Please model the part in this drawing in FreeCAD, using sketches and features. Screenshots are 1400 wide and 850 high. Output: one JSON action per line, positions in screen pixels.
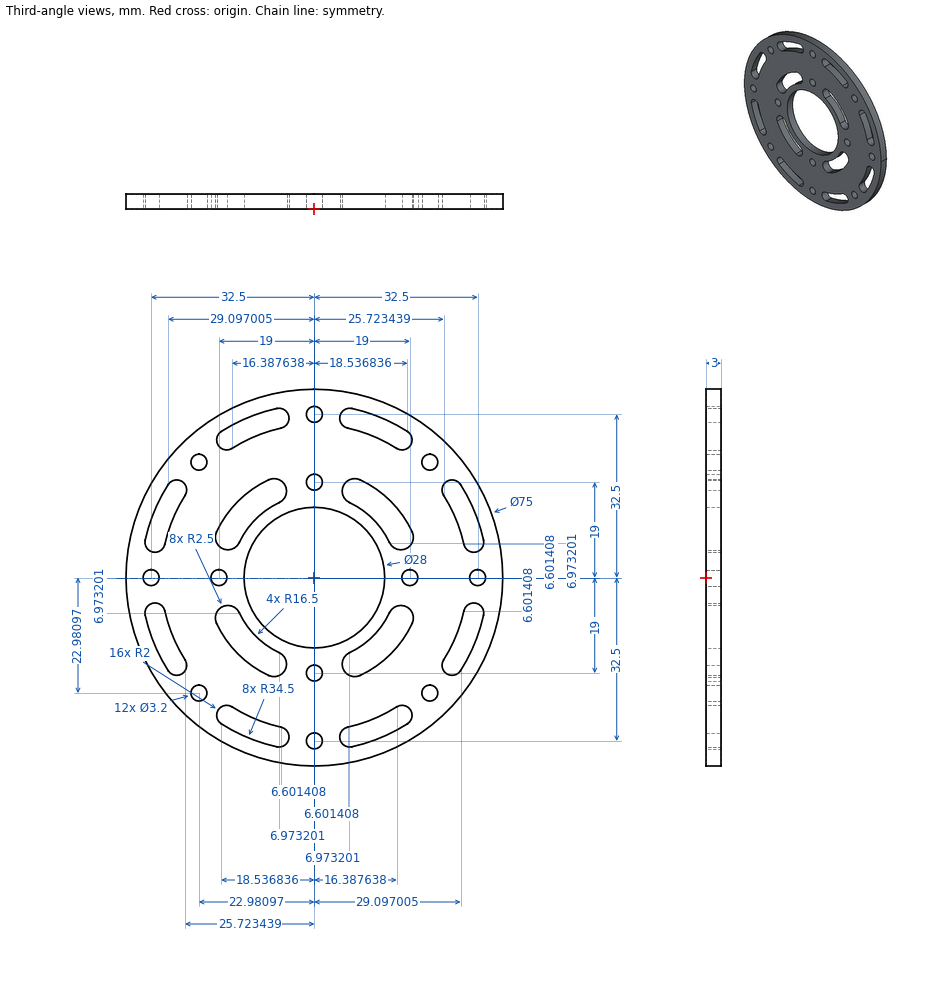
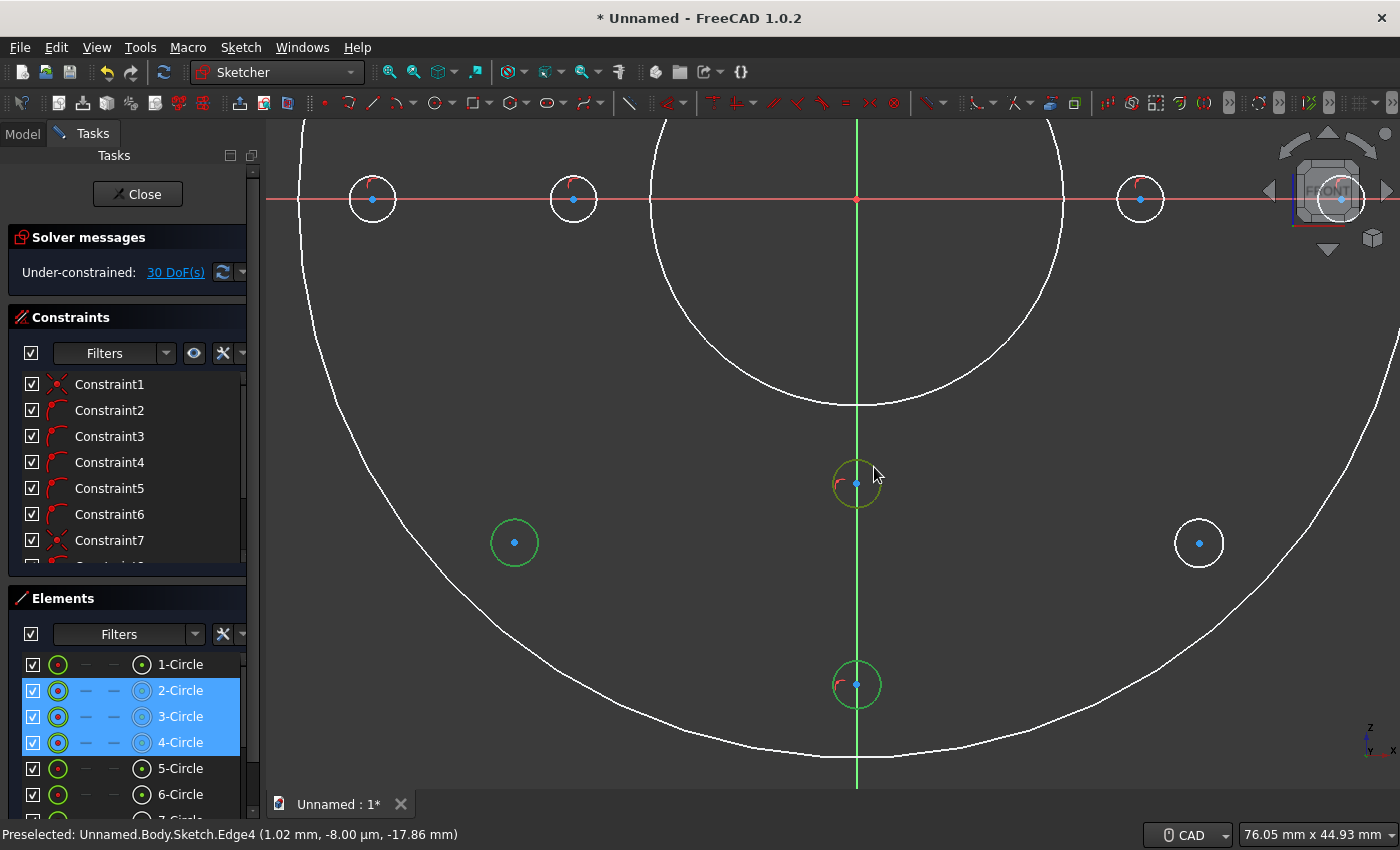
{"action": "left_click", "coordinate": [389, 183]}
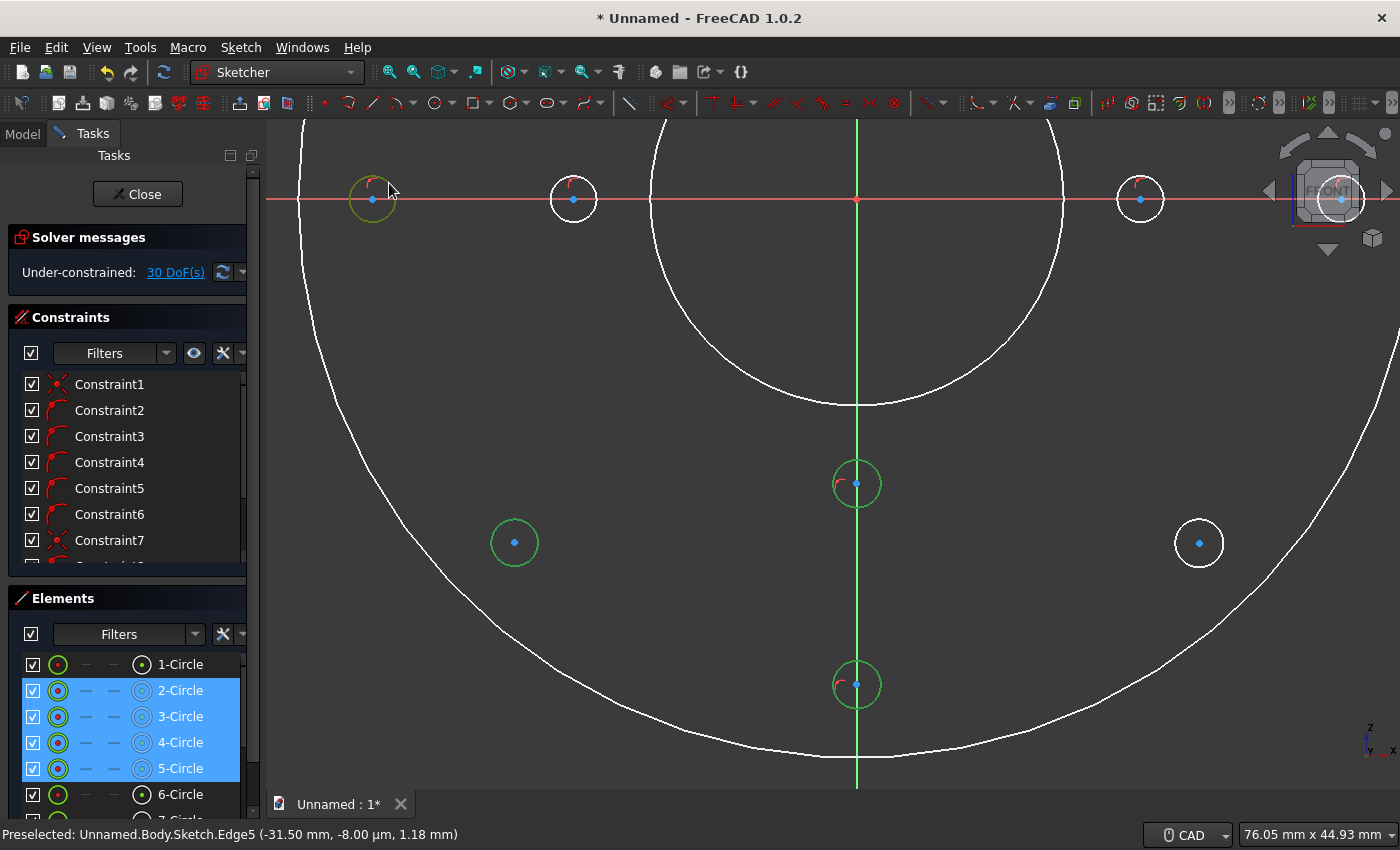
{"action": "left_click", "coordinate": [590, 183]}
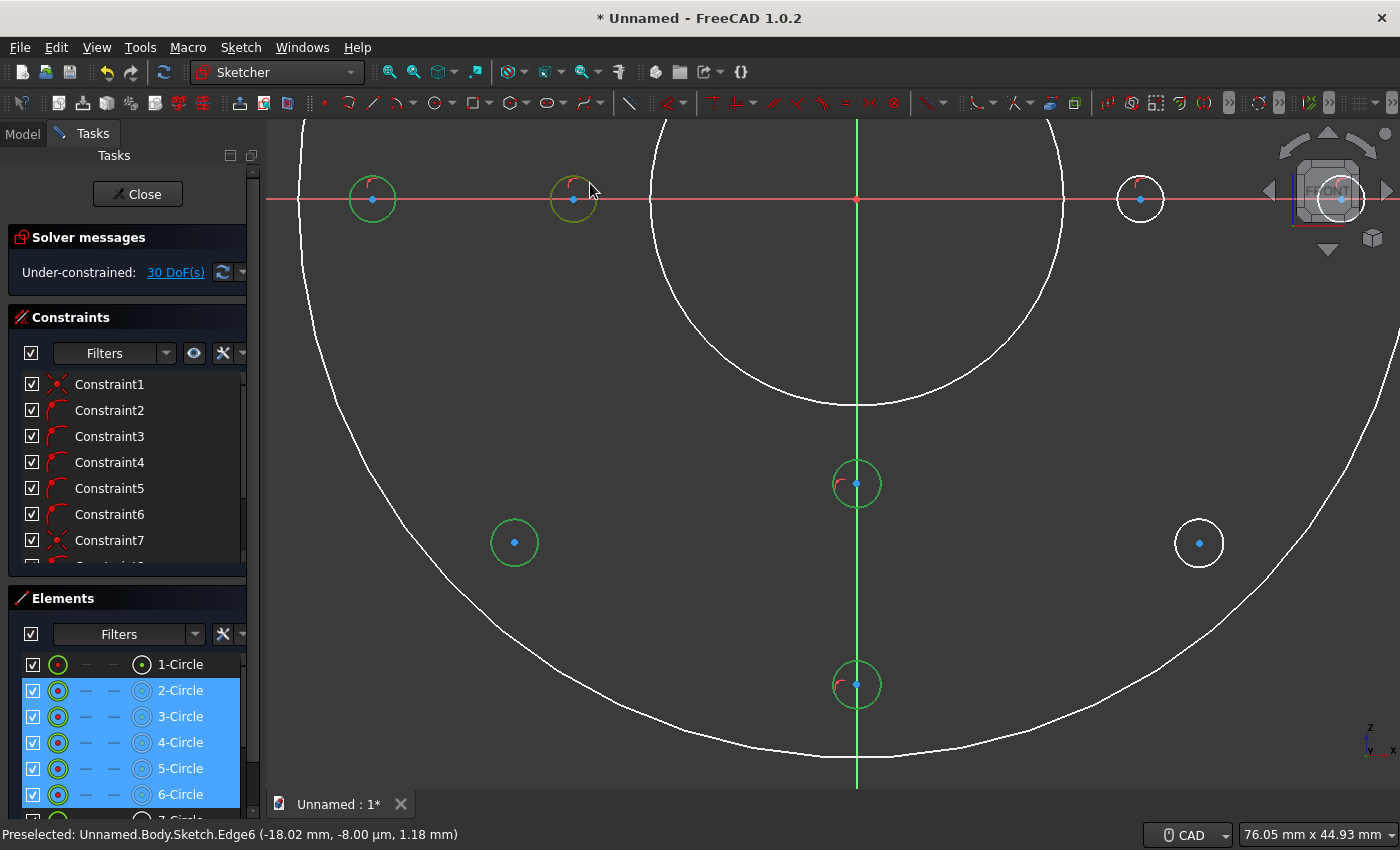
{"action": "scroll", "coordinate": [711, 602], "scroll_direction": "down", "scroll_amount": 5}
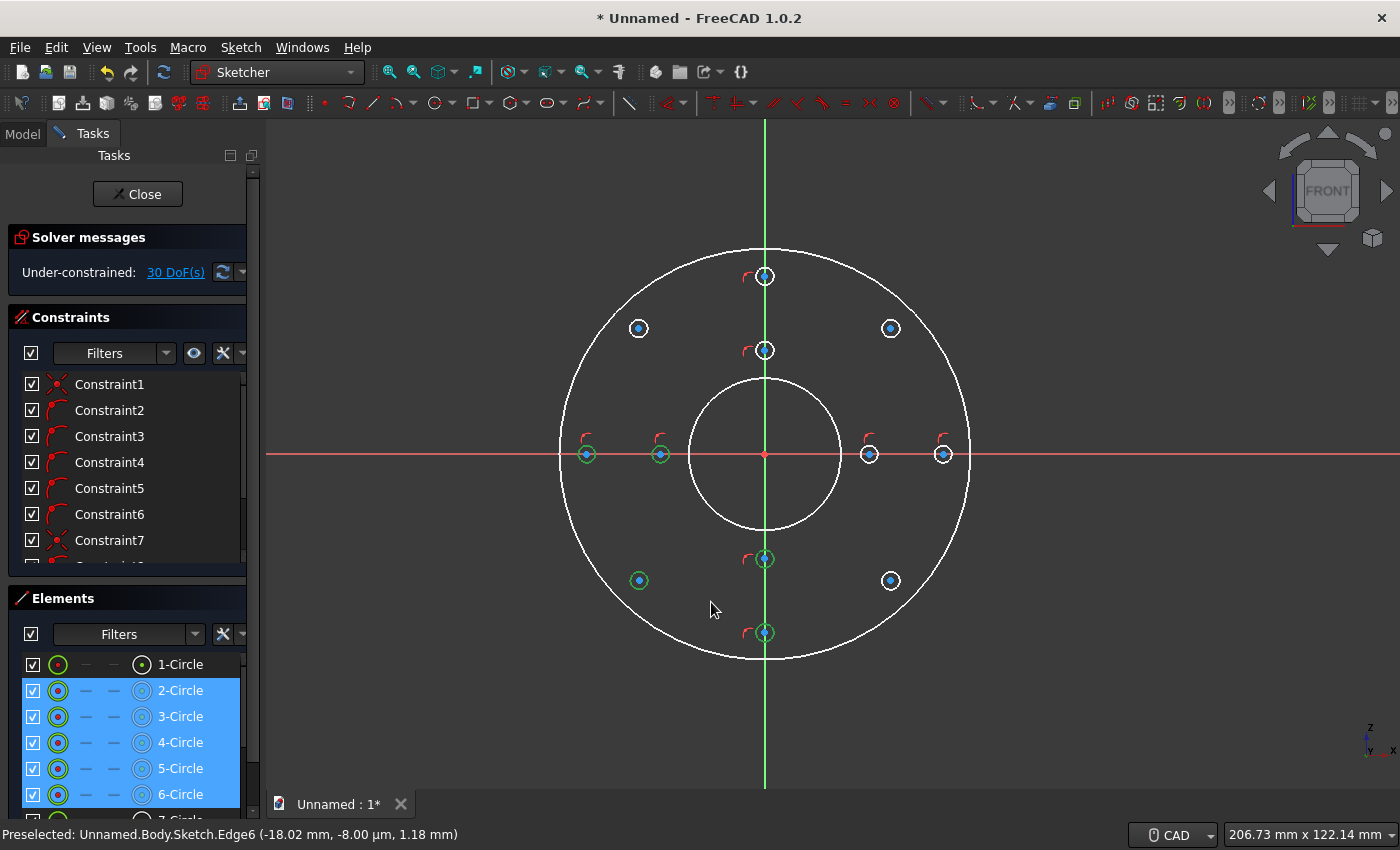
{"action": "scroll", "coordinate": [645, 322], "scroll_direction": "up", "scroll_amount": 3}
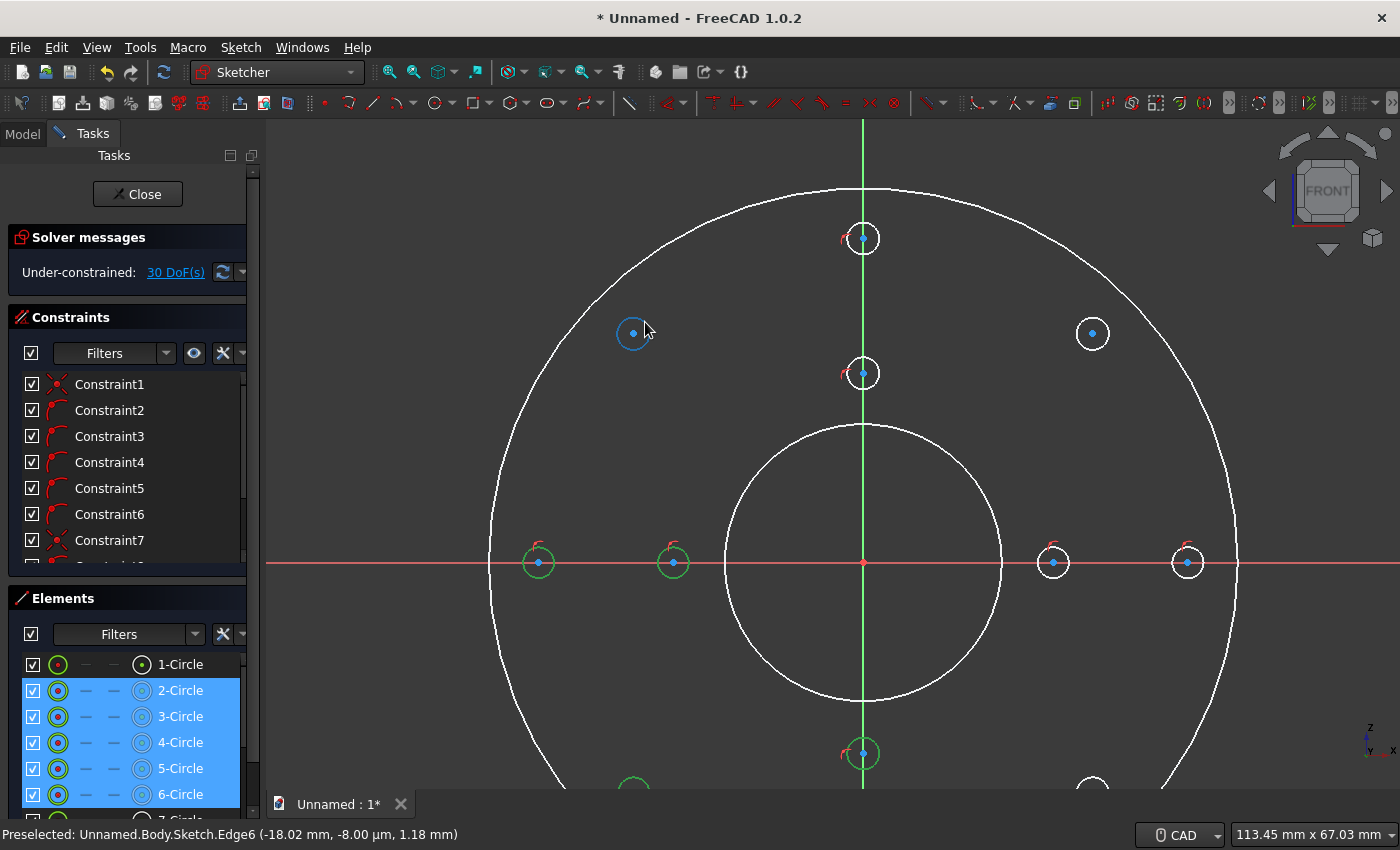
{"action": "left_click", "coordinate": [645, 322]}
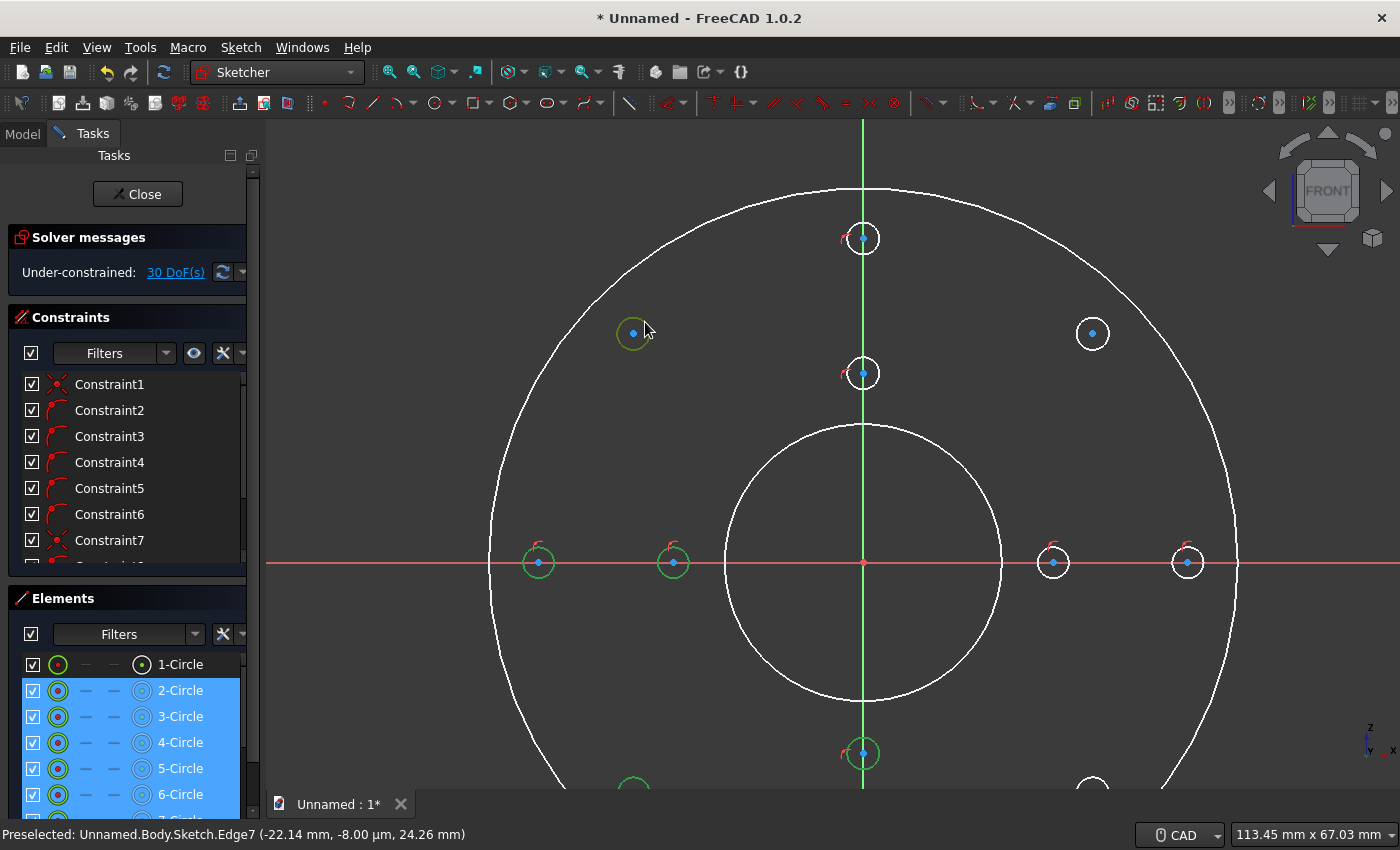
{"action": "scroll", "coordinate": [644, 322], "scroll_direction": "down", "scroll_amount": 3}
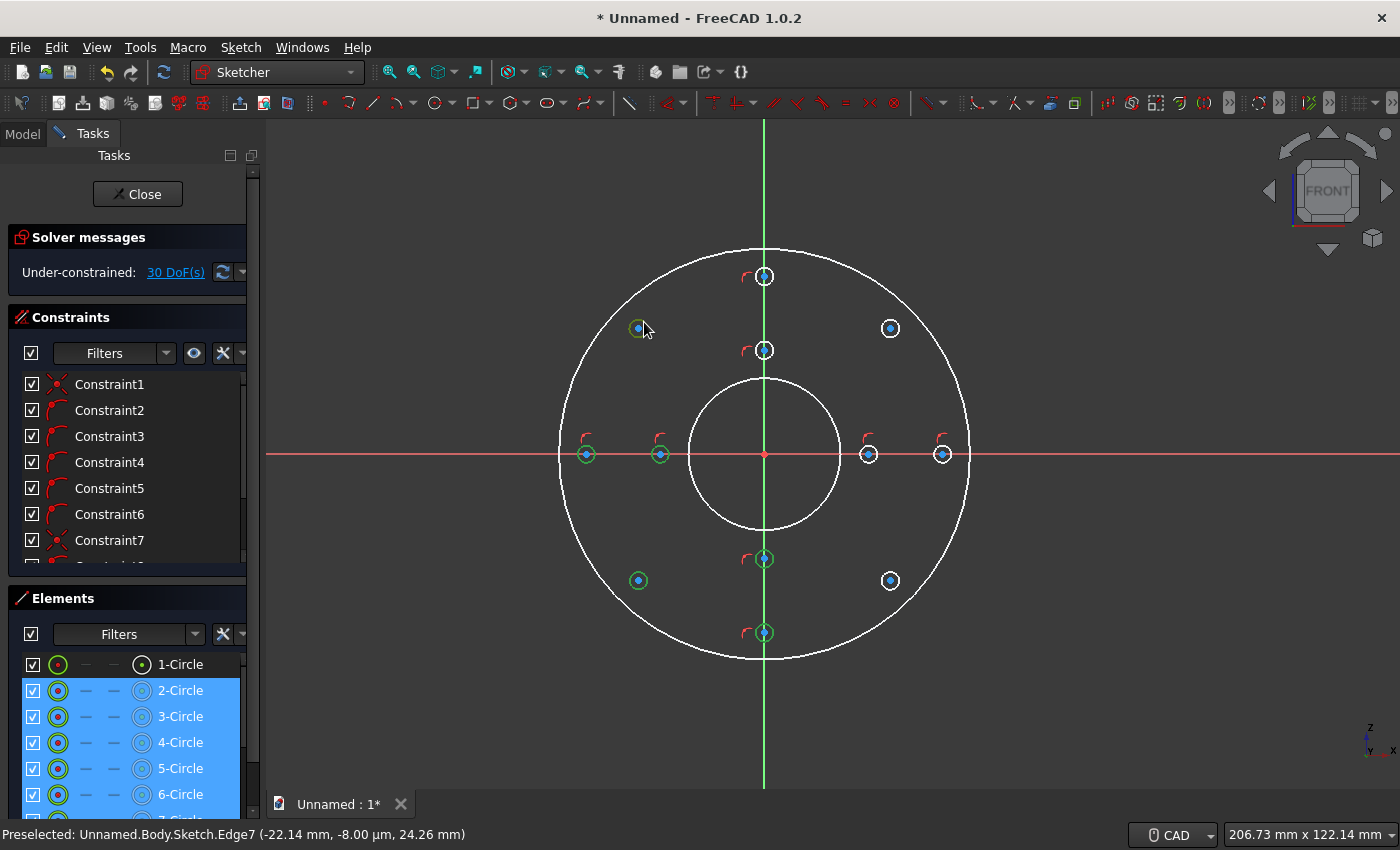
{"action": "scroll", "coordinate": [897, 575], "scroll_direction": "up", "scroll_amount": 3}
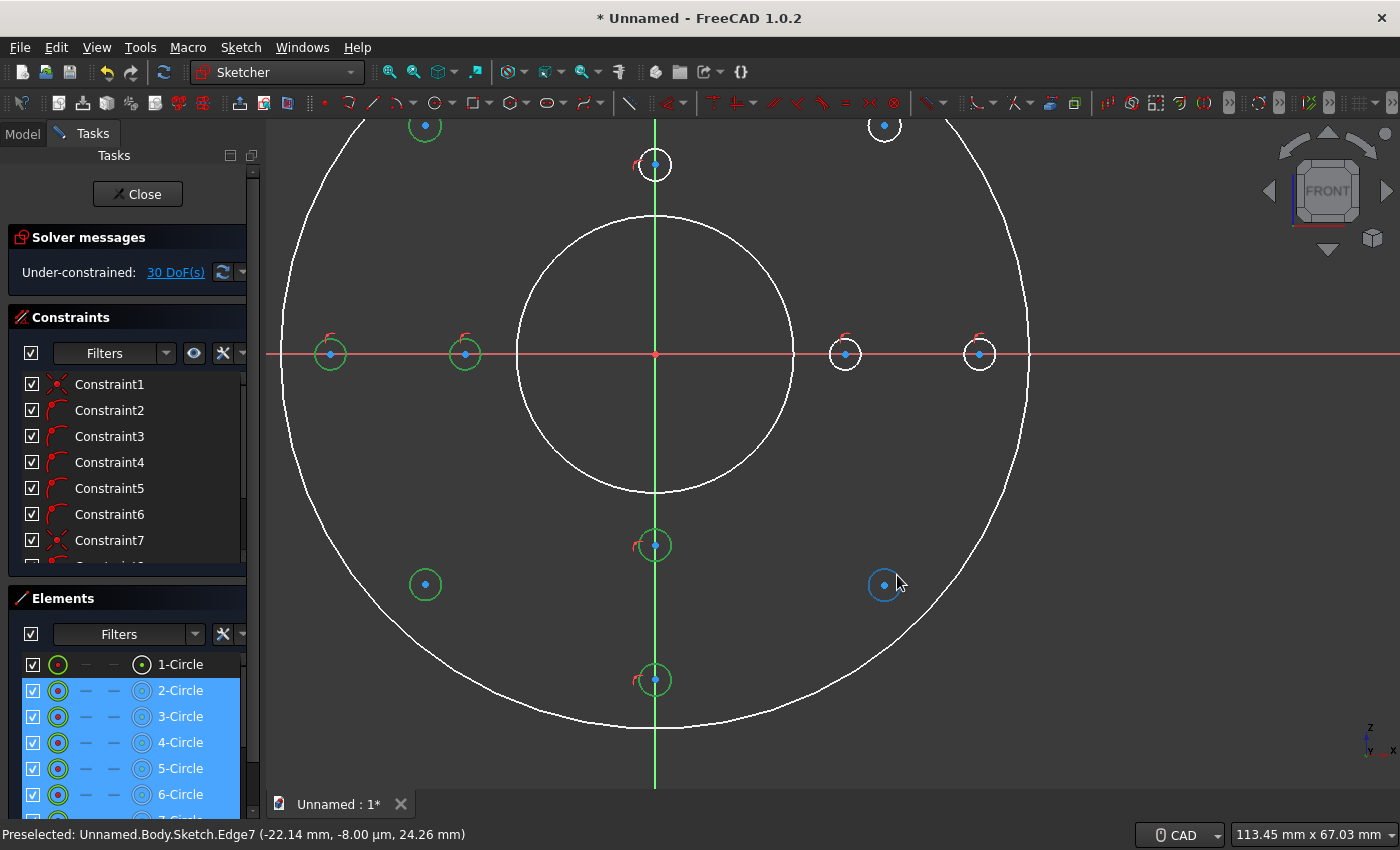
{"action": "left_click", "coordinate": [896, 574]}